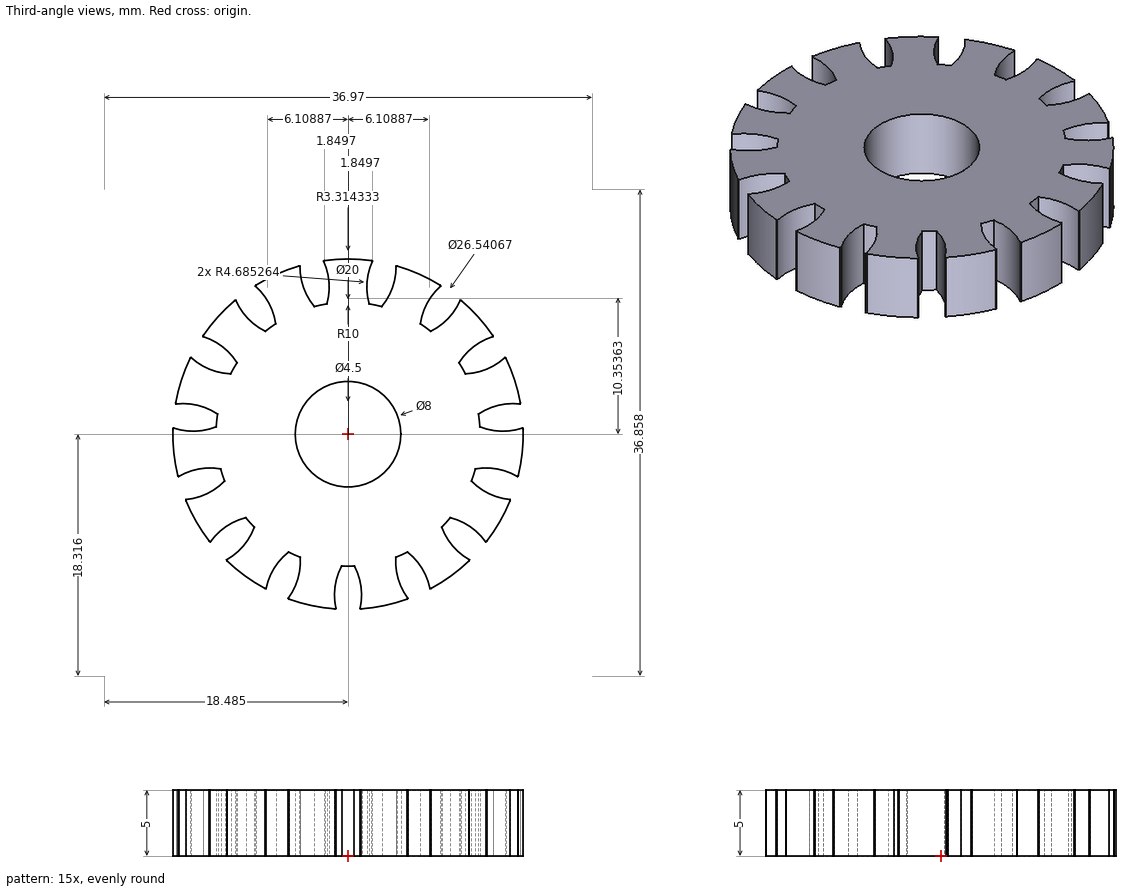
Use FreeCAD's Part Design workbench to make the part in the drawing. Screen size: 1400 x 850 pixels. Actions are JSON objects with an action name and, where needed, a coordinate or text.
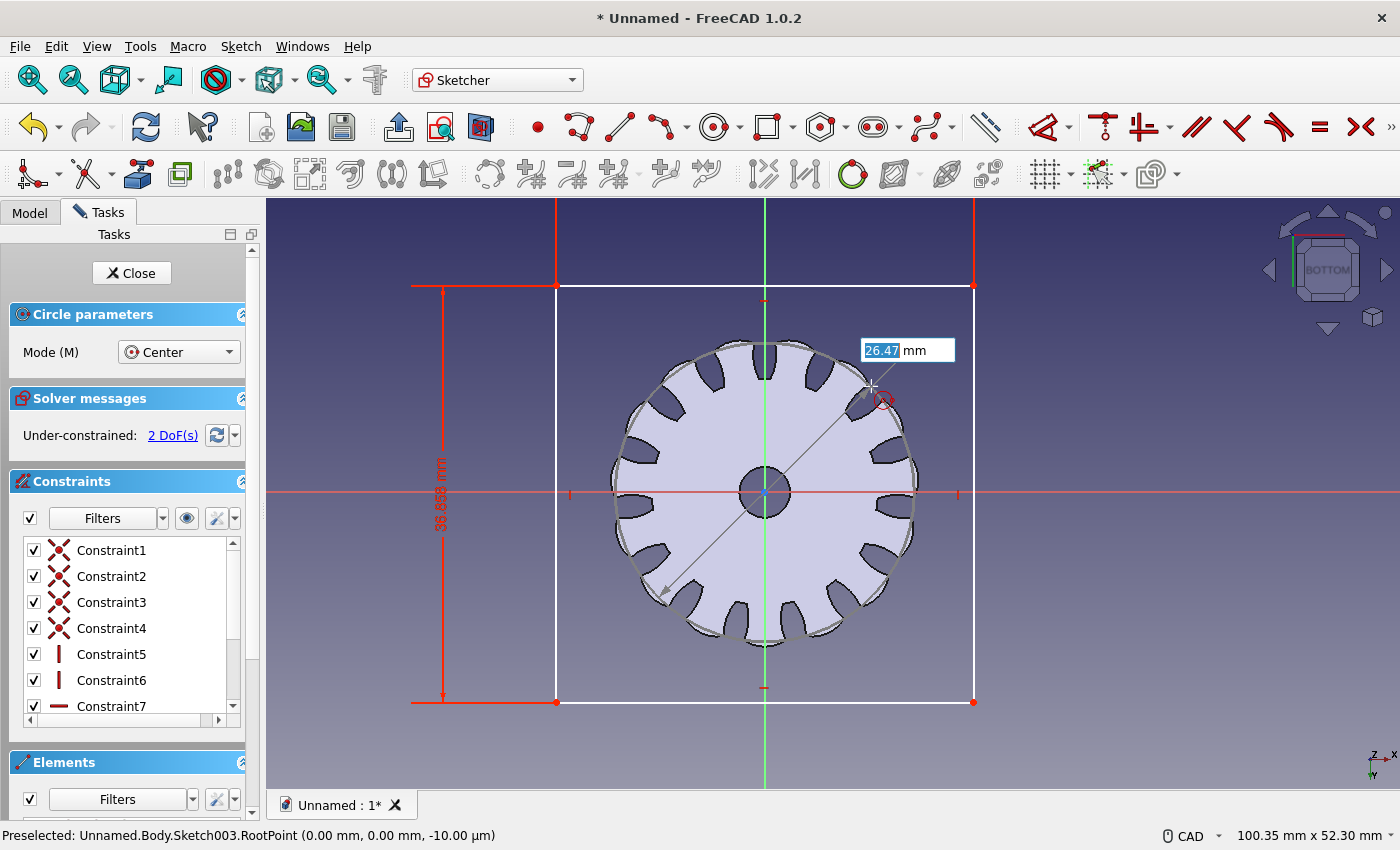
{"action": "type", "text": "26.54067"}
{"action": "key", "text": "Return"}
{"action": "key", "text": "Escape"}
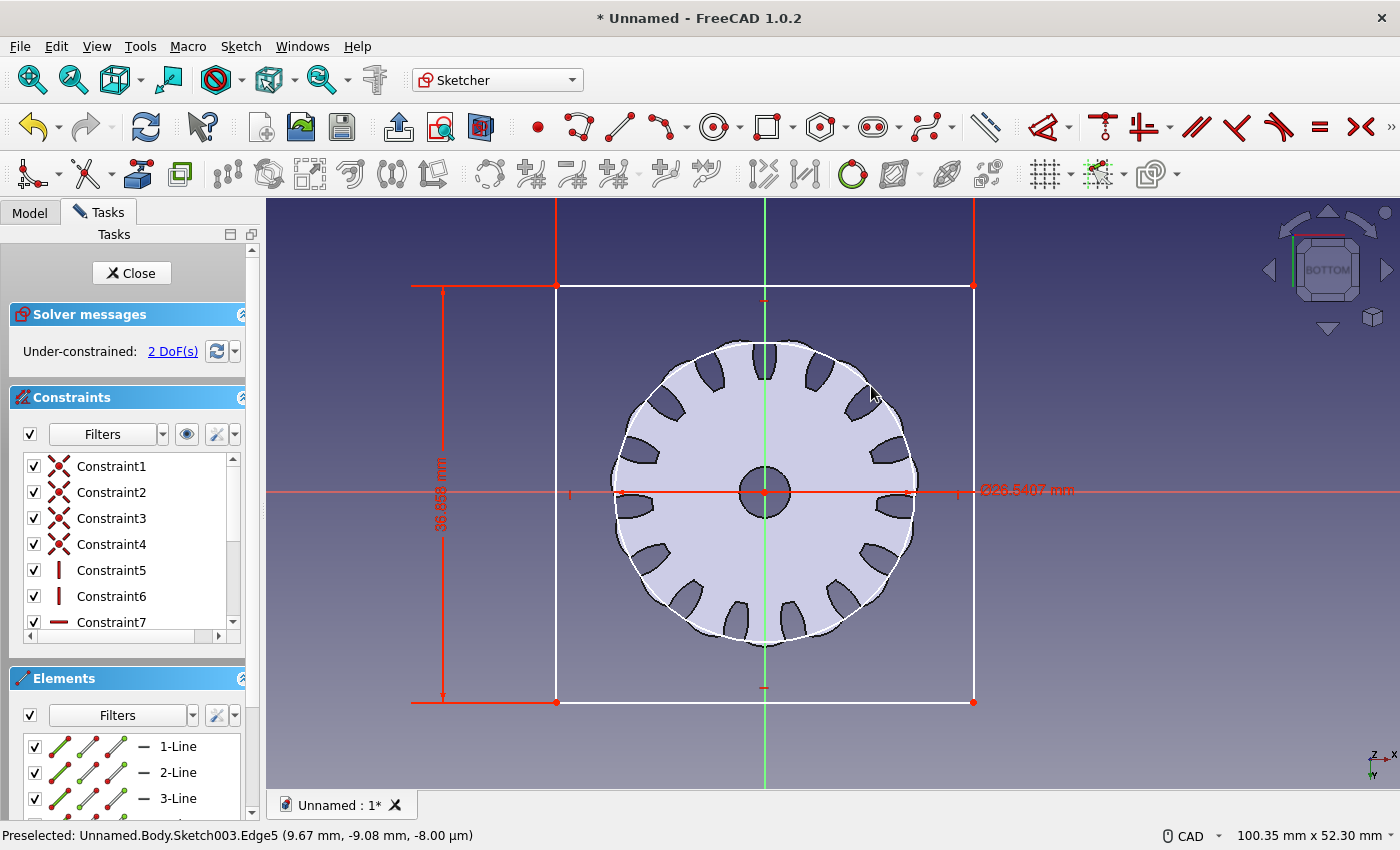
{"action": "key", "text": "d"}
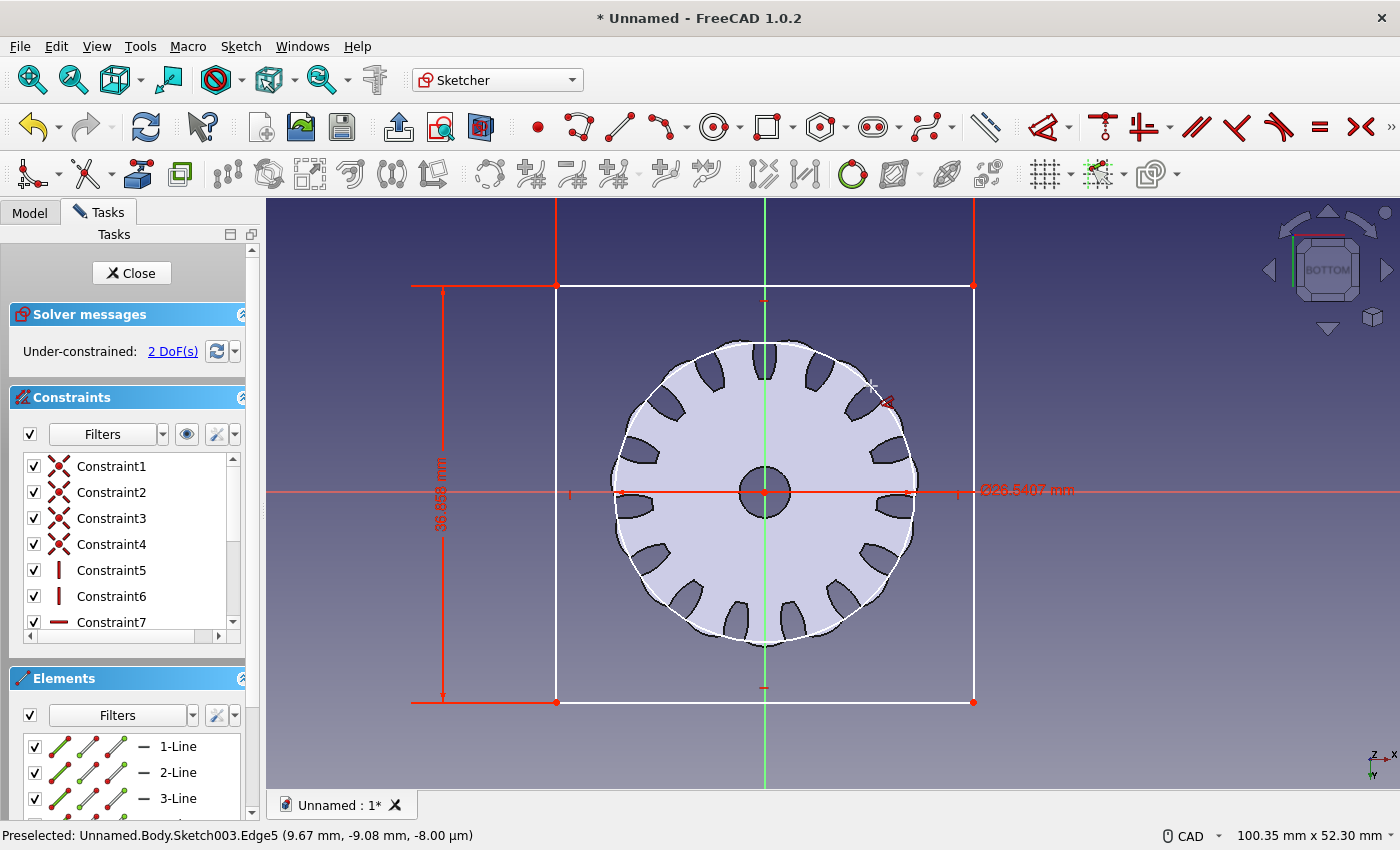
{"action": "left_click", "coordinate": [556, 286]}
{"action": "left_click", "coordinate": [660, 252]}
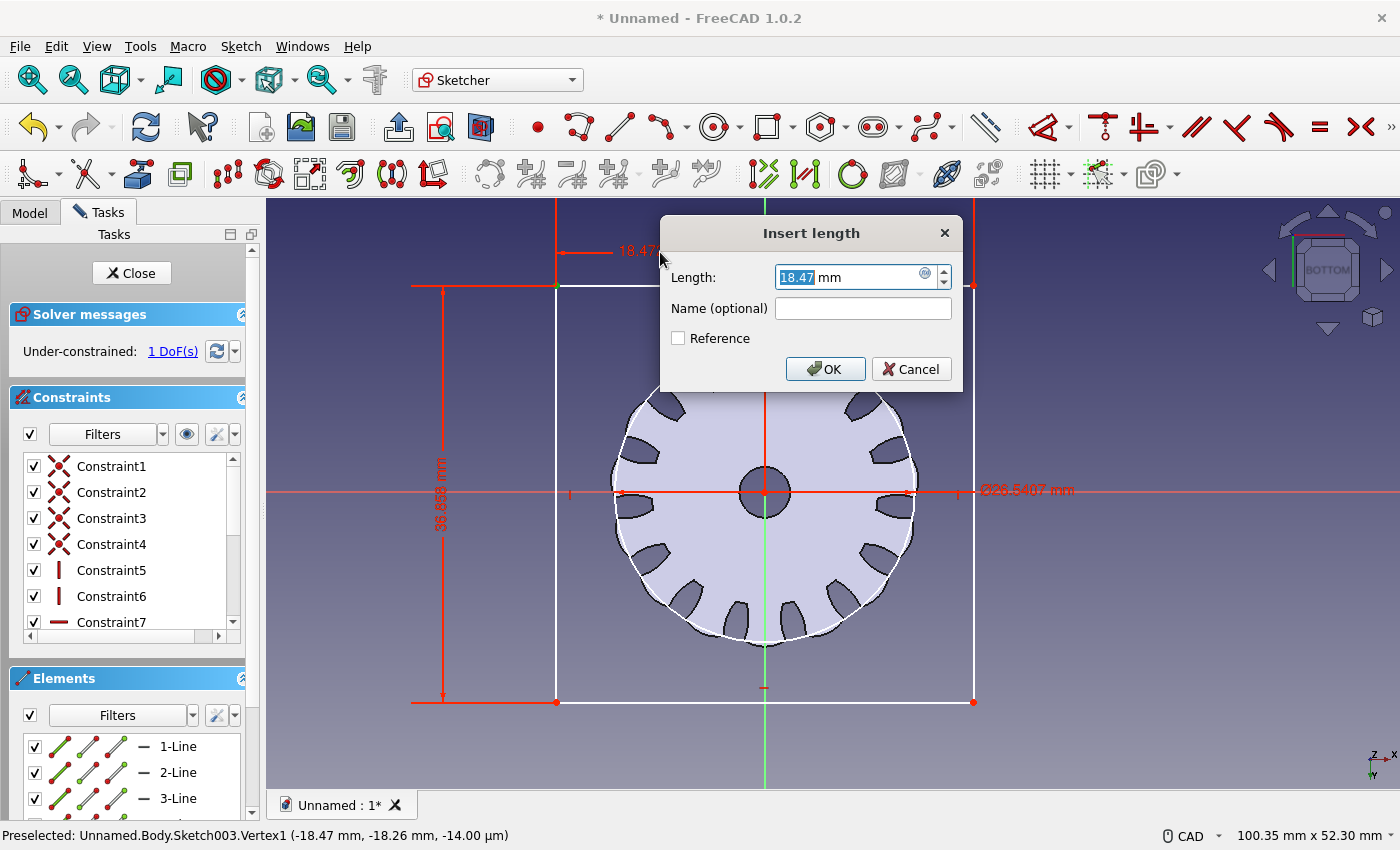
{"action": "type", "text": "18.485"}
{"action": "key", "text": "Return"}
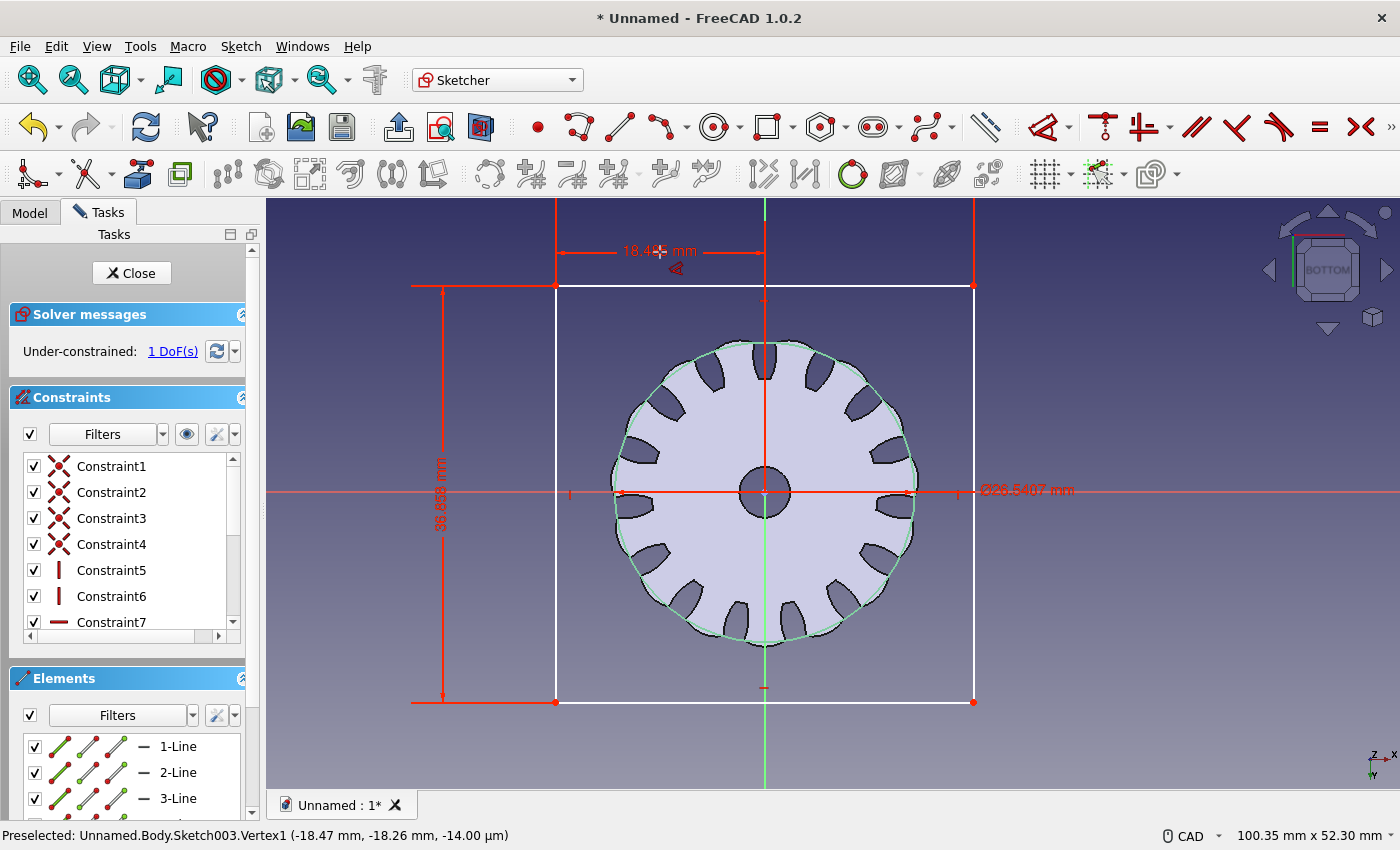
{"action": "left_click", "coordinate": [556, 286]}
{"action": "left_click", "coordinate": [522, 389]}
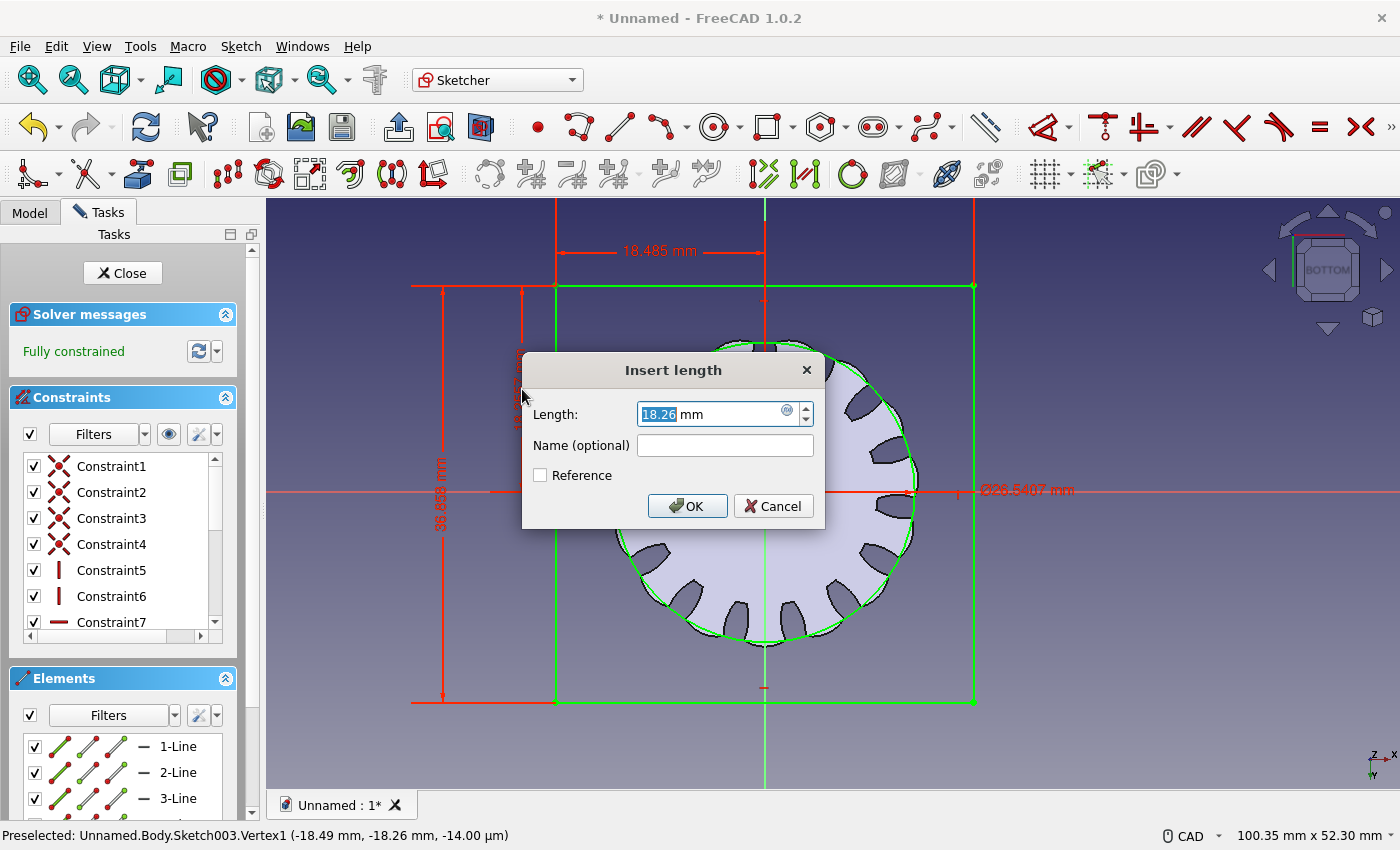
{"action": "type", "text": "18.316"}
{"action": "key", "text": "Return"}
{"action": "key", "text": "Escape"}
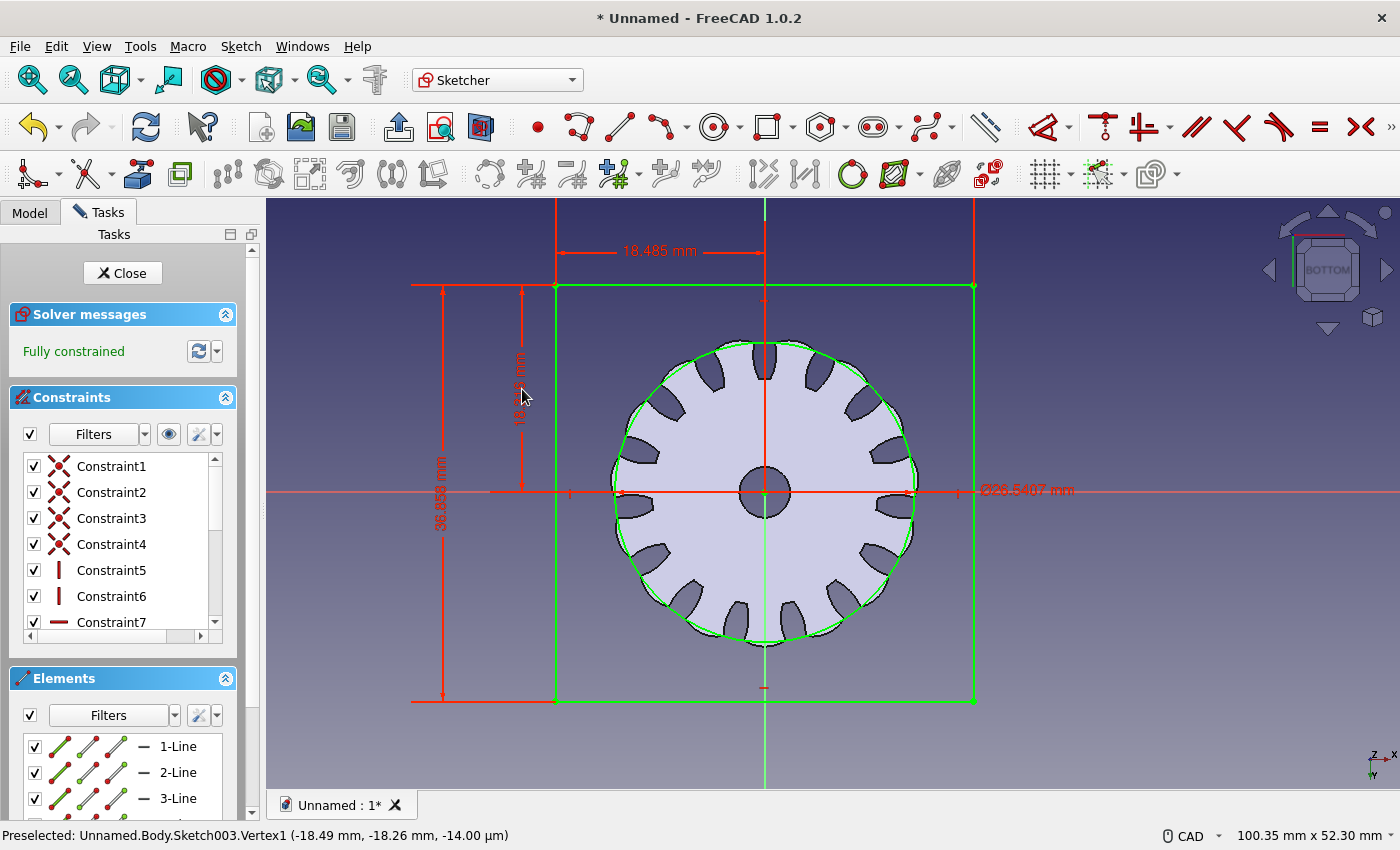
{"action": "left_click", "coordinate": [123, 273]}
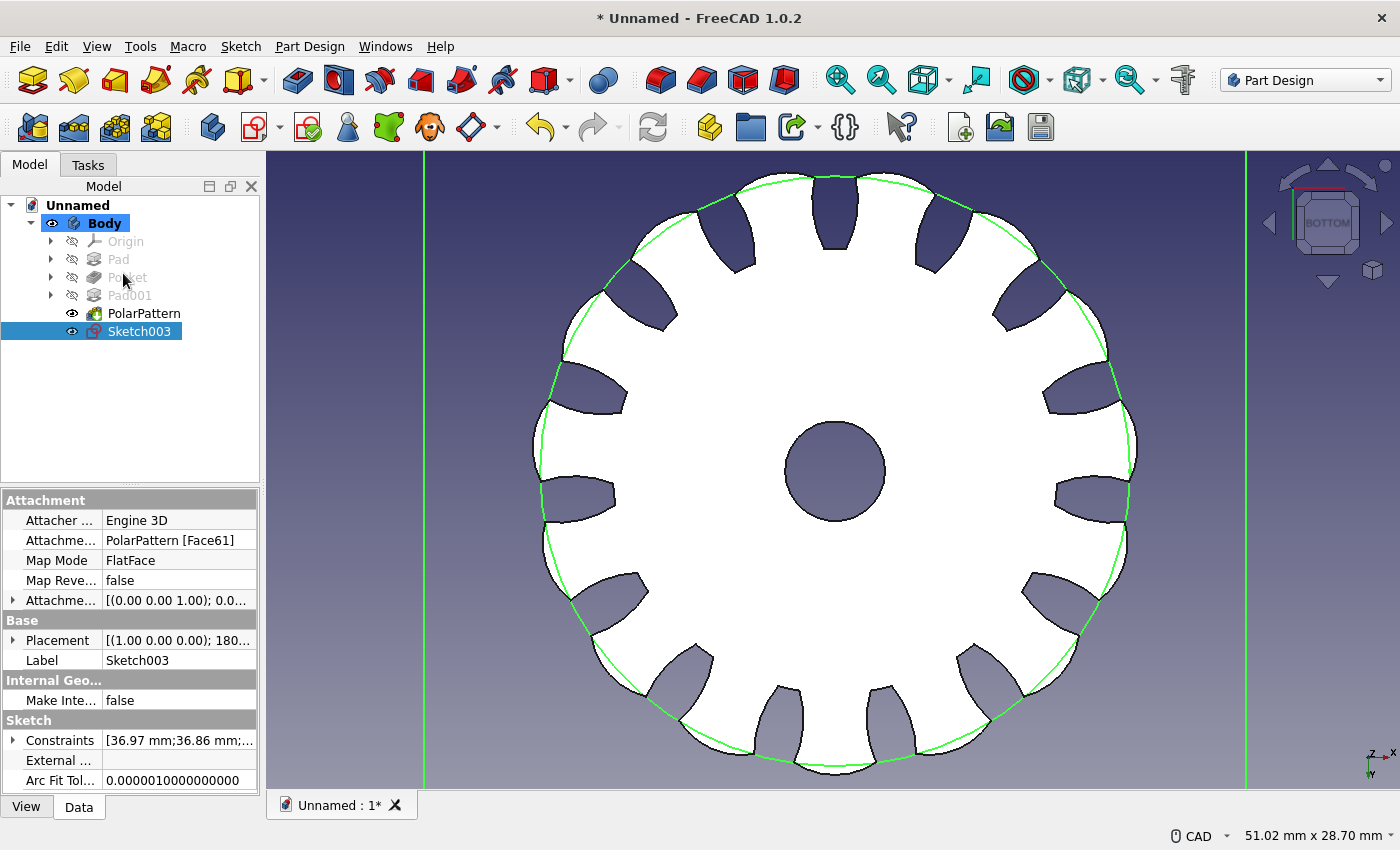
{"action": "left_click", "coordinate": [298, 80]}